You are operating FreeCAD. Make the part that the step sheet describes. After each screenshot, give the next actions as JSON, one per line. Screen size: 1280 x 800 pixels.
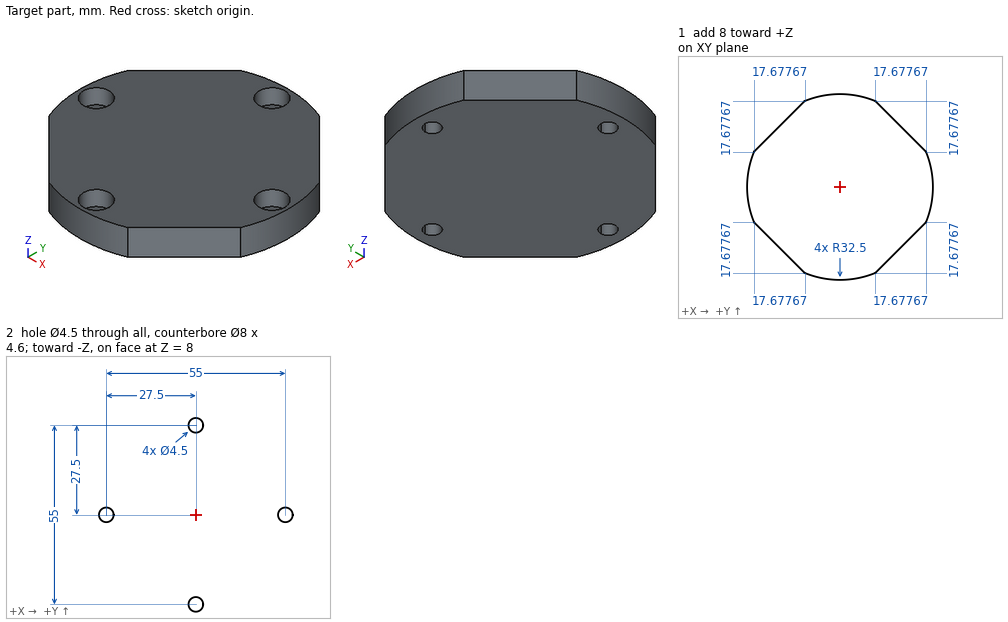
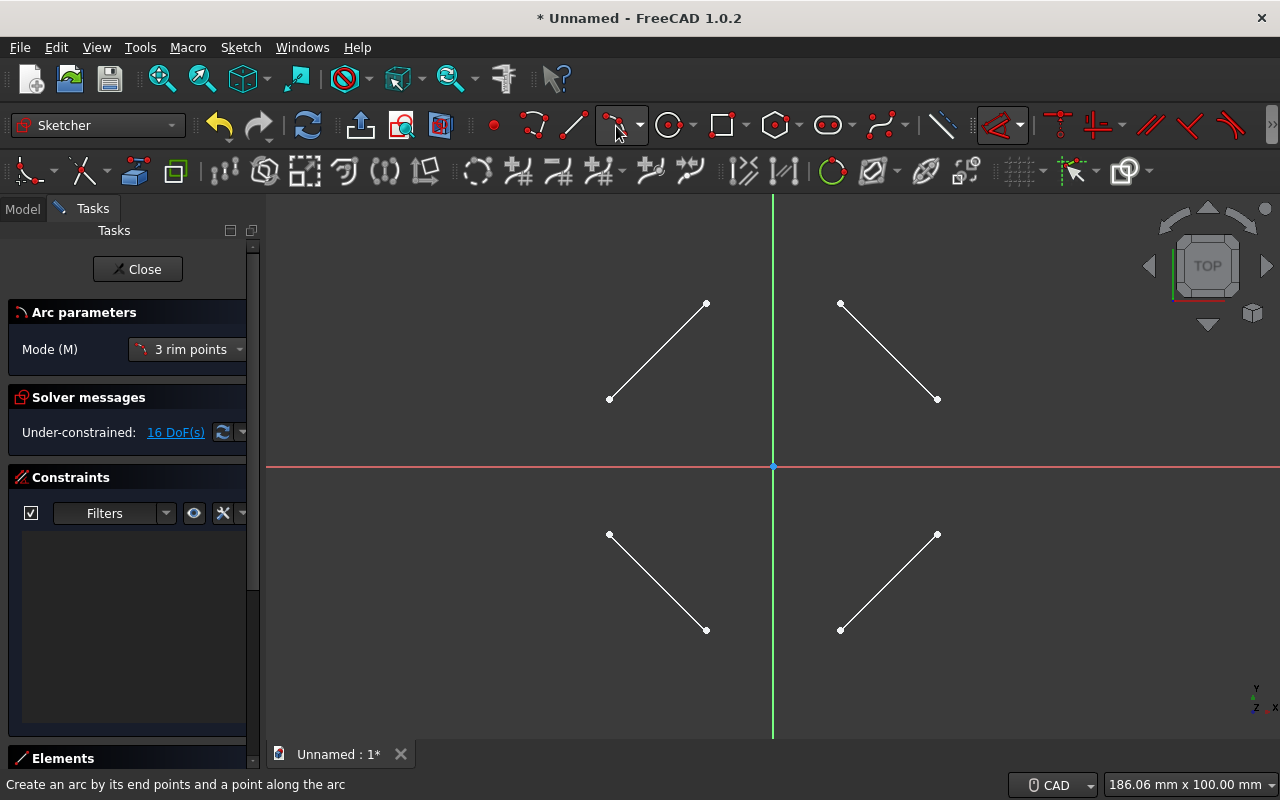
{"action": "left_click", "coordinate": [706, 631]}
{"action": "left_click", "coordinate": [840, 631]}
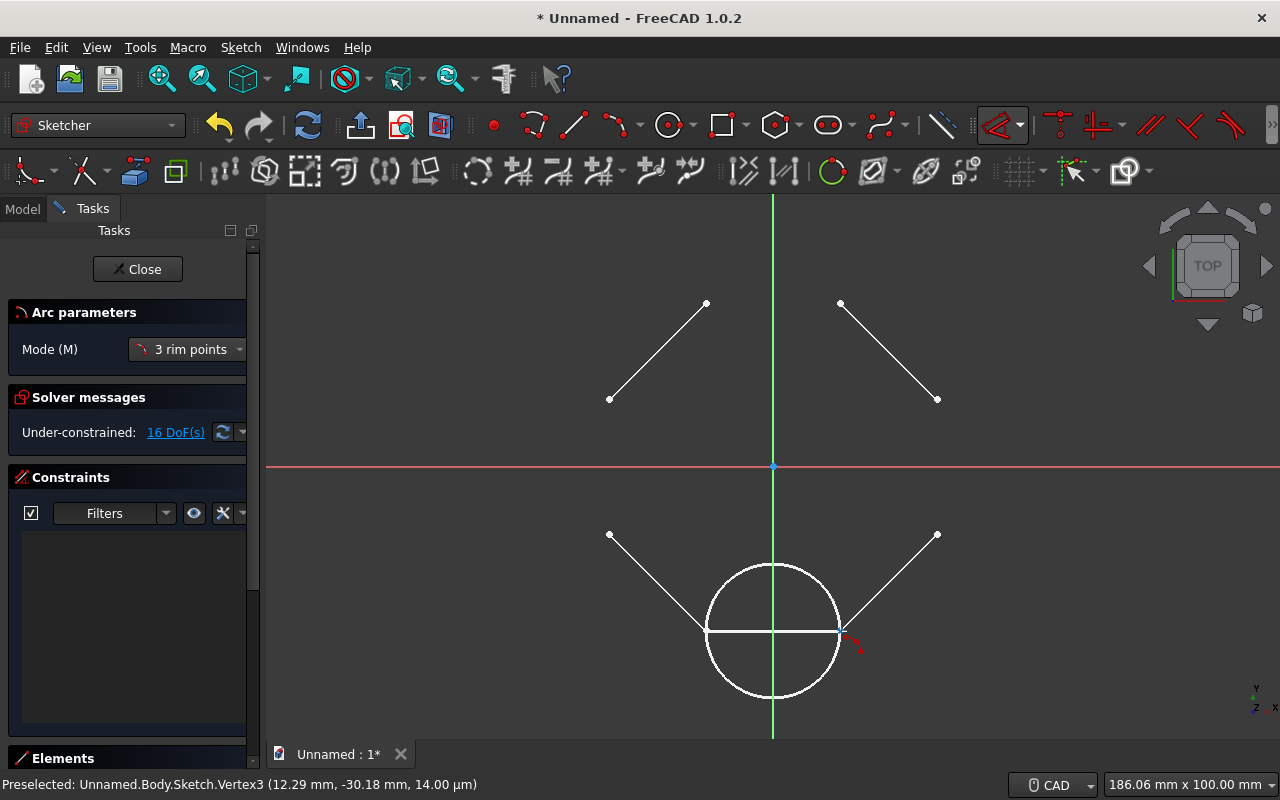
{"action": "scroll", "coordinate": [759, 643], "scroll_direction": "up", "scroll_amount": 2}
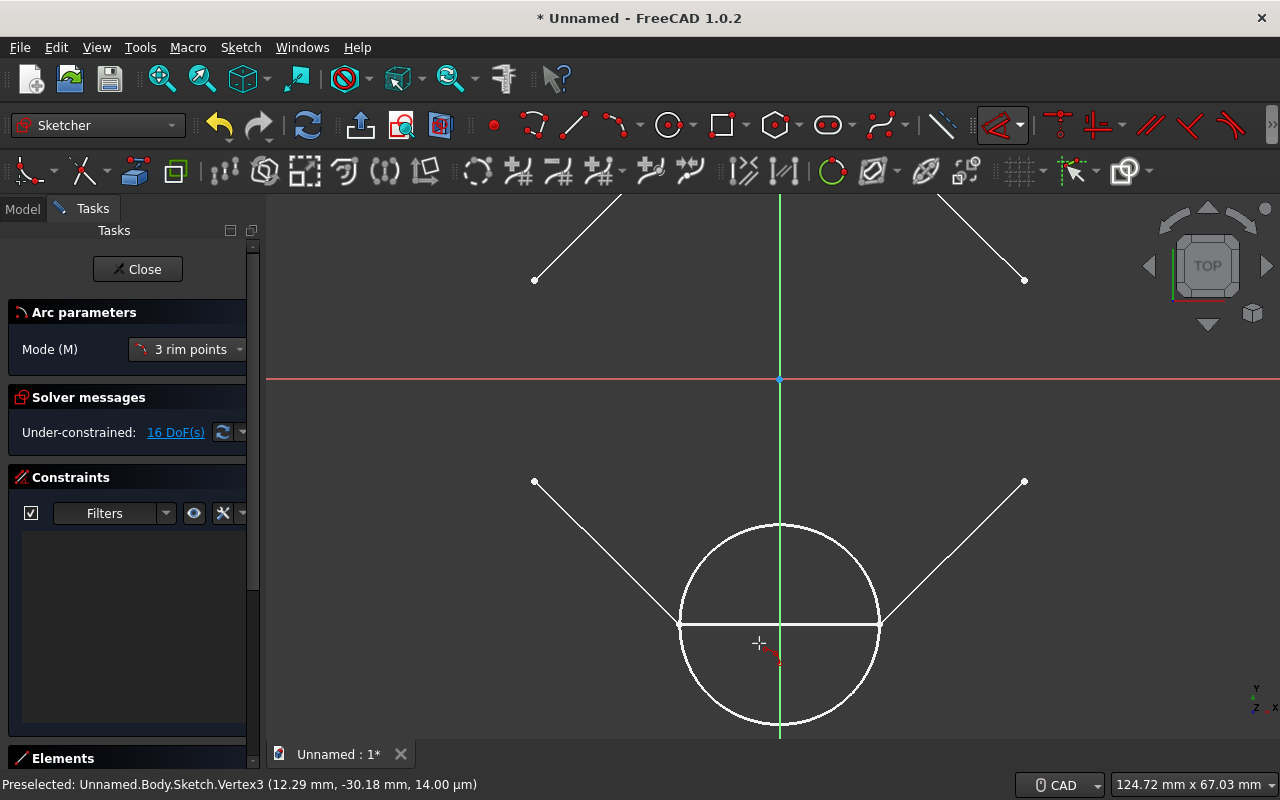
{"action": "left_click", "coordinate": [759, 643]}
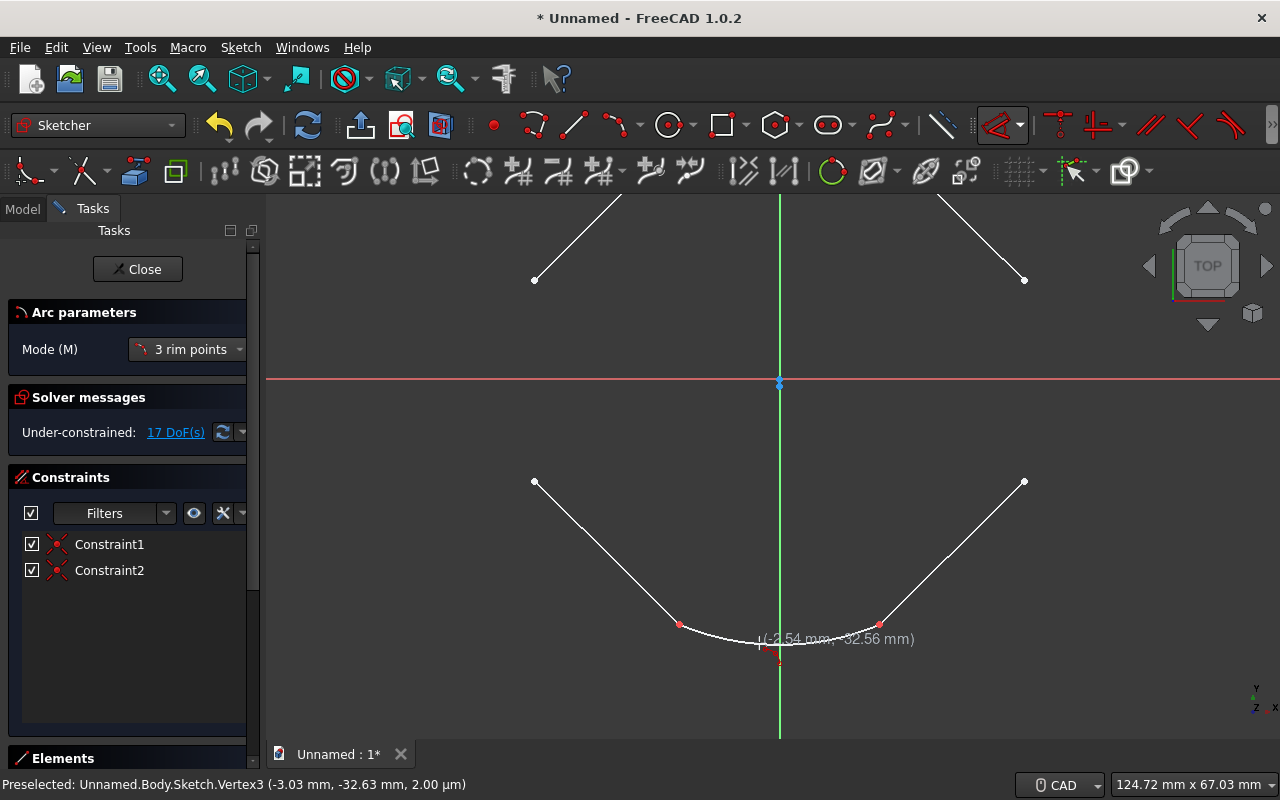
{"action": "left_click", "coordinate": [1024, 481]}
{"action": "left_click", "coordinate": [1024, 280]}
{"action": "left_click", "coordinate": [1043, 400]}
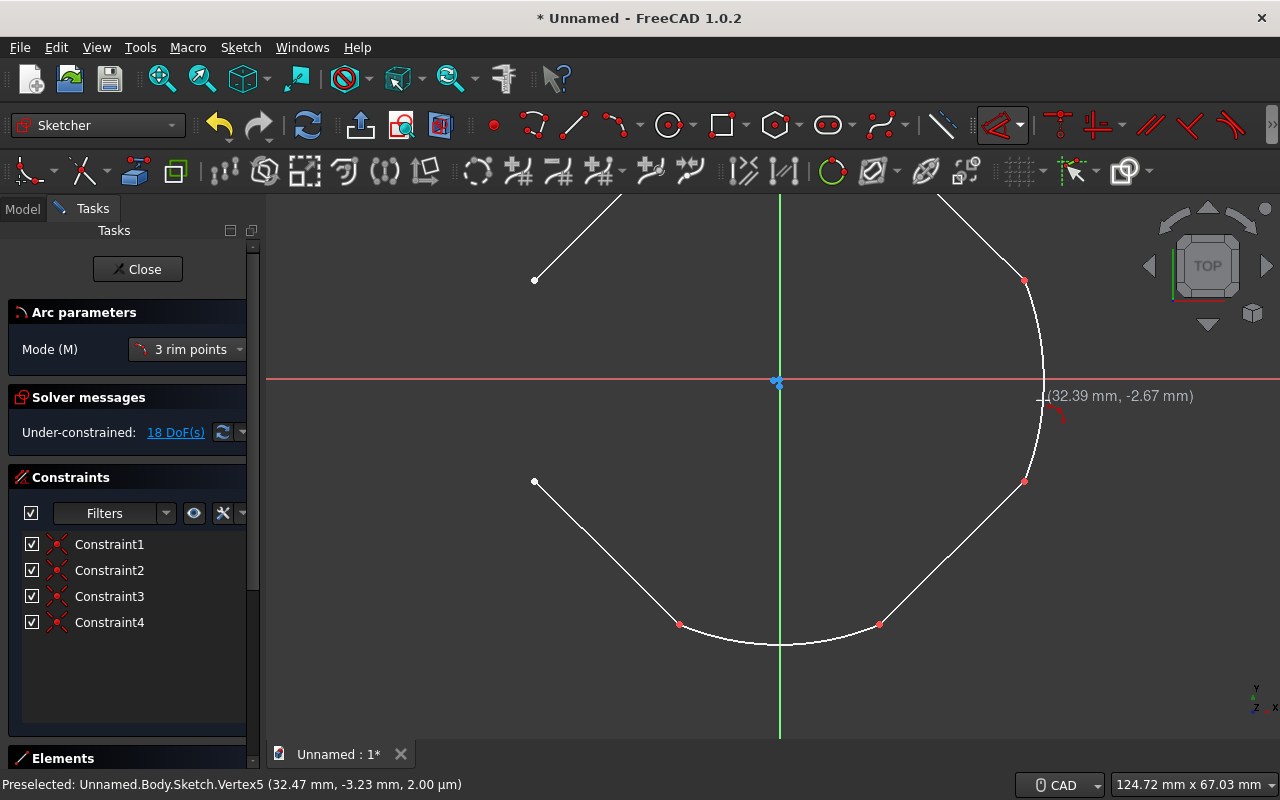
{"action": "scroll", "coordinate": [552, 644], "scroll_direction": "down", "scroll_amount": 2}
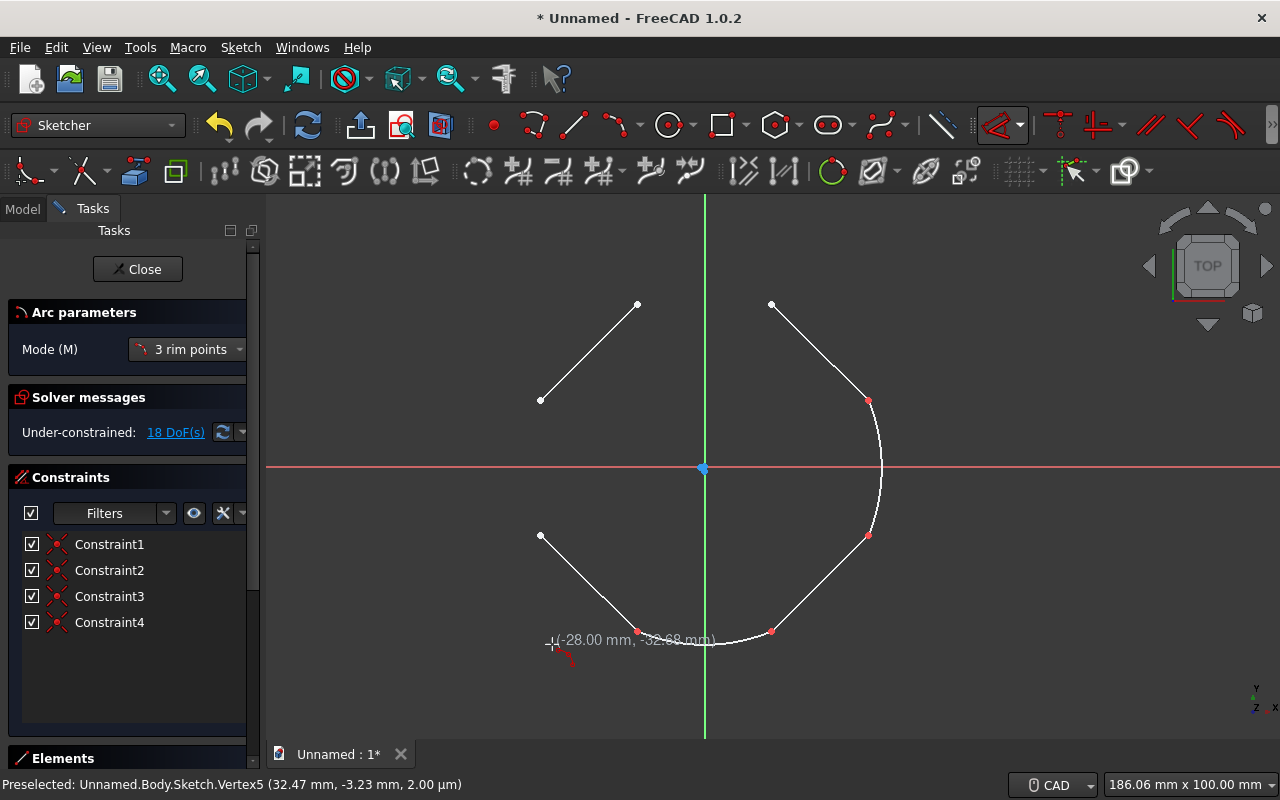
{"action": "left_click", "coordinate": [772, 304]}
{"action": "left_click", "coordinate": [638, 304]}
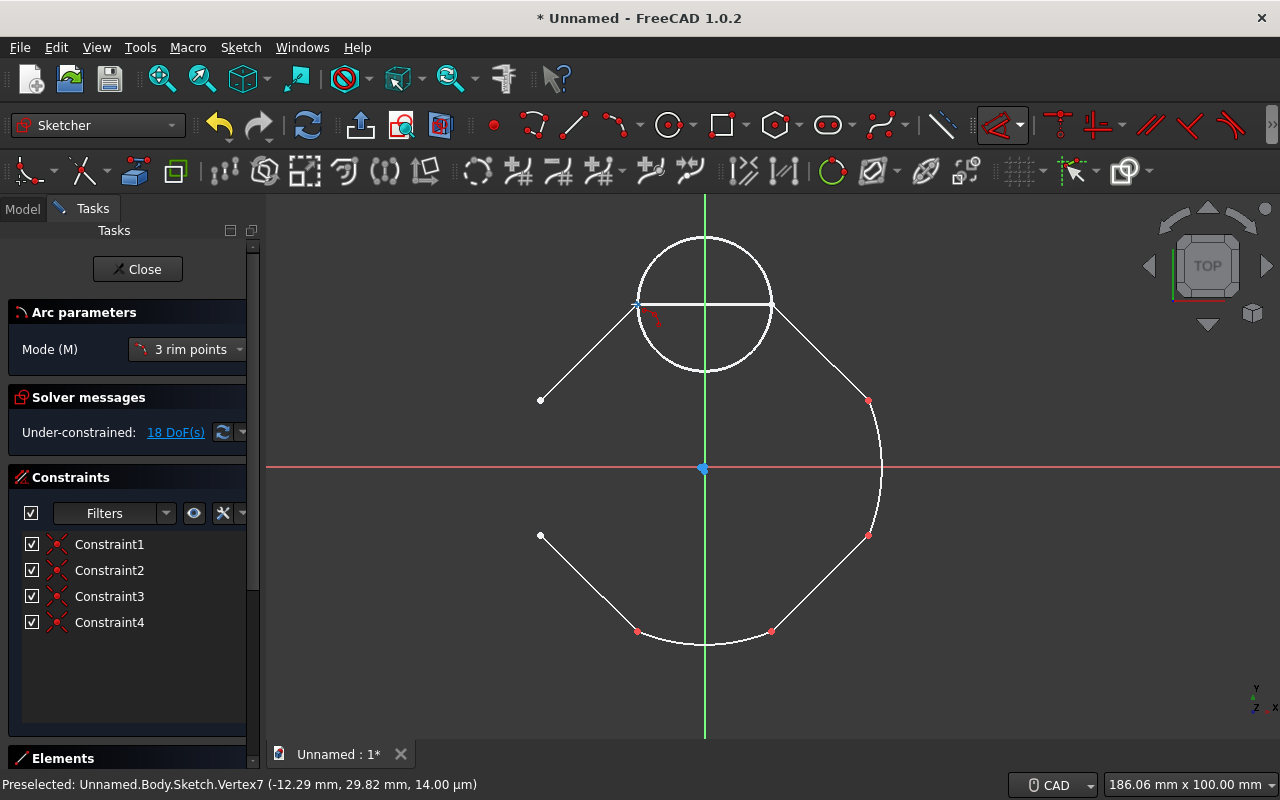
{"action": "scroll", "coordinate": [719, 290], "scroll_direction": "up", "scroll_amount": 2}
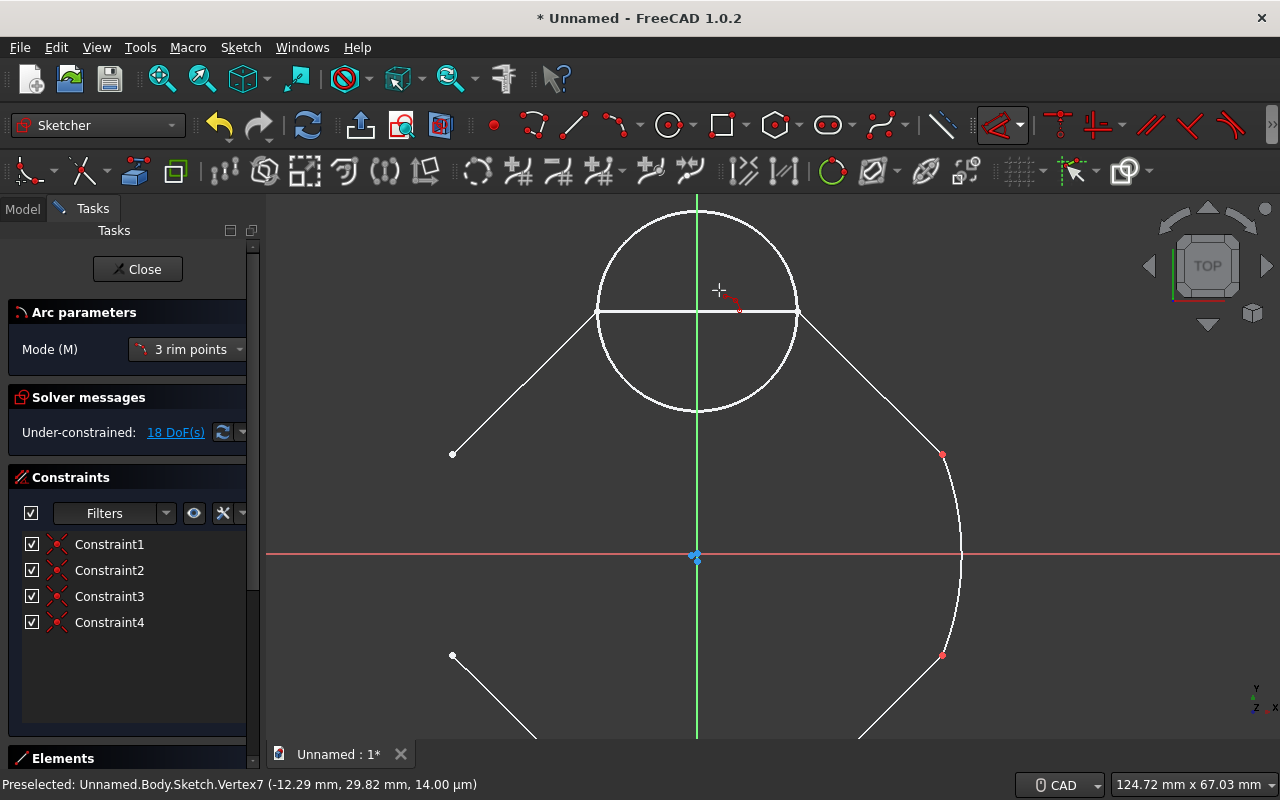
{"action": "left_click", "coordinate": [718, 290]}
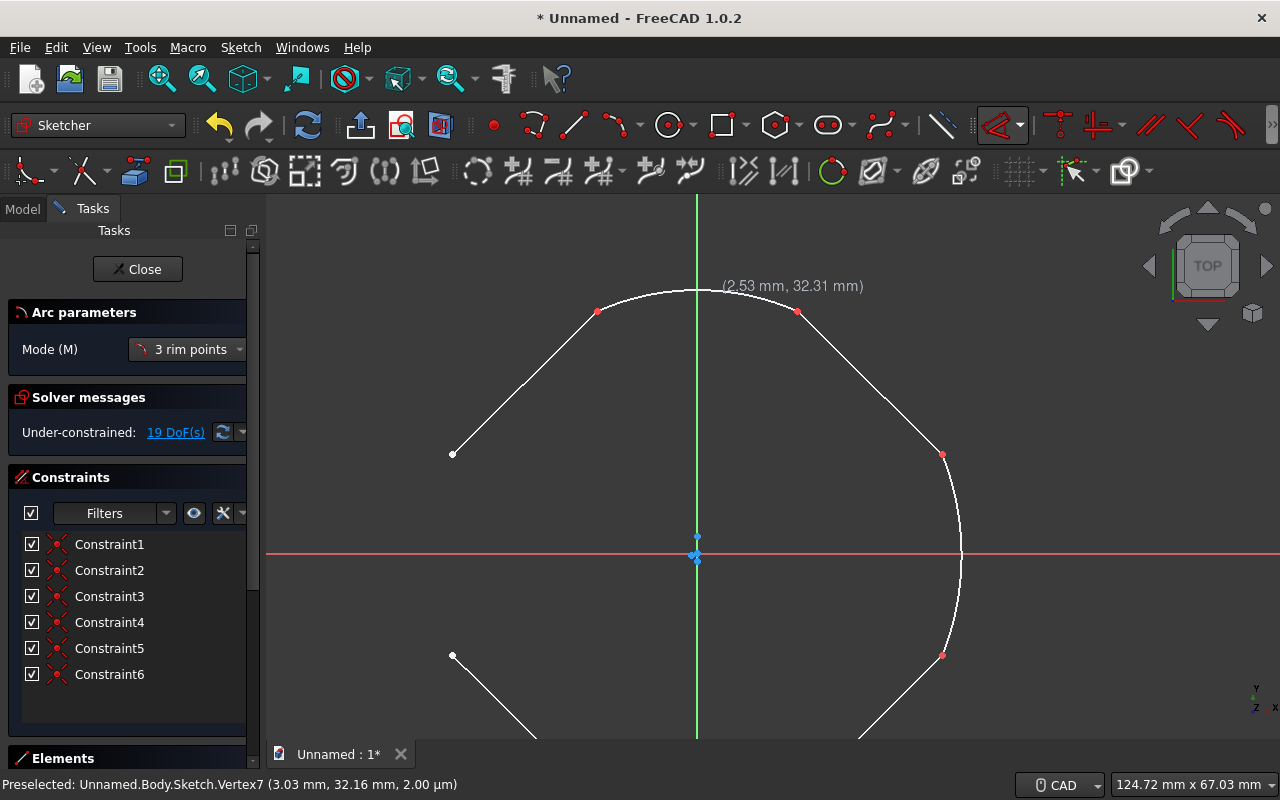
{"action": "left_click", "coordinate": [453, 455]}
{"action": "left_click", "coordinate": [453, 656]}
{"action": "left_click", "coordinate": [434, 533]}
{"action": "key", "text": "Escape"}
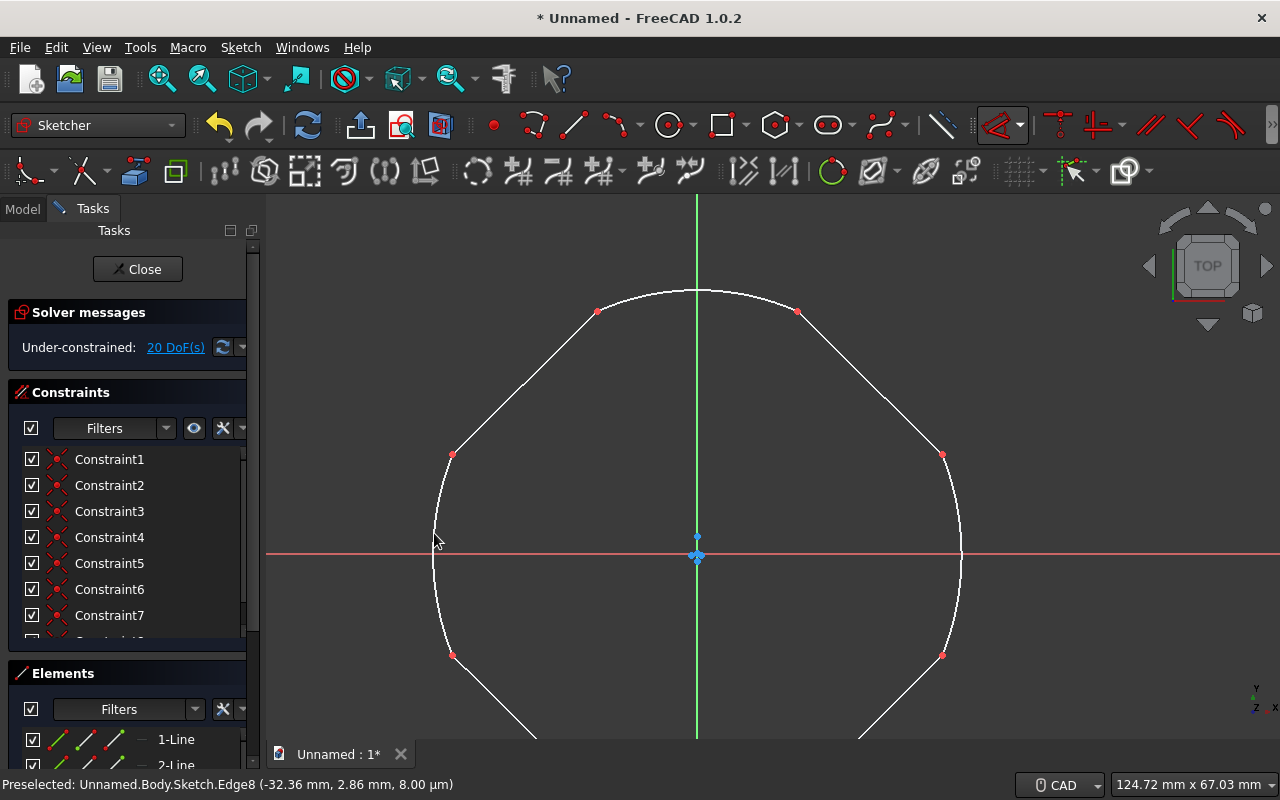
{"action": "scroll", "coordinate": [719, 289], "scroll_direction": "down", "scroll_amount": 2}